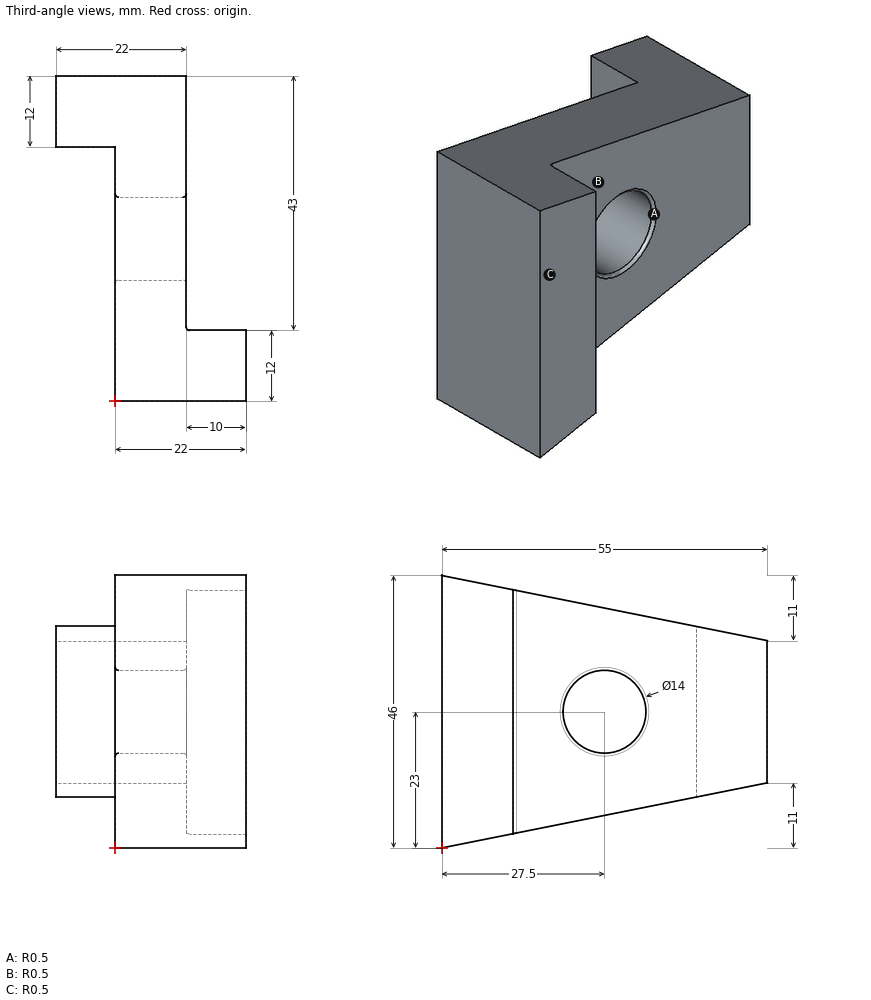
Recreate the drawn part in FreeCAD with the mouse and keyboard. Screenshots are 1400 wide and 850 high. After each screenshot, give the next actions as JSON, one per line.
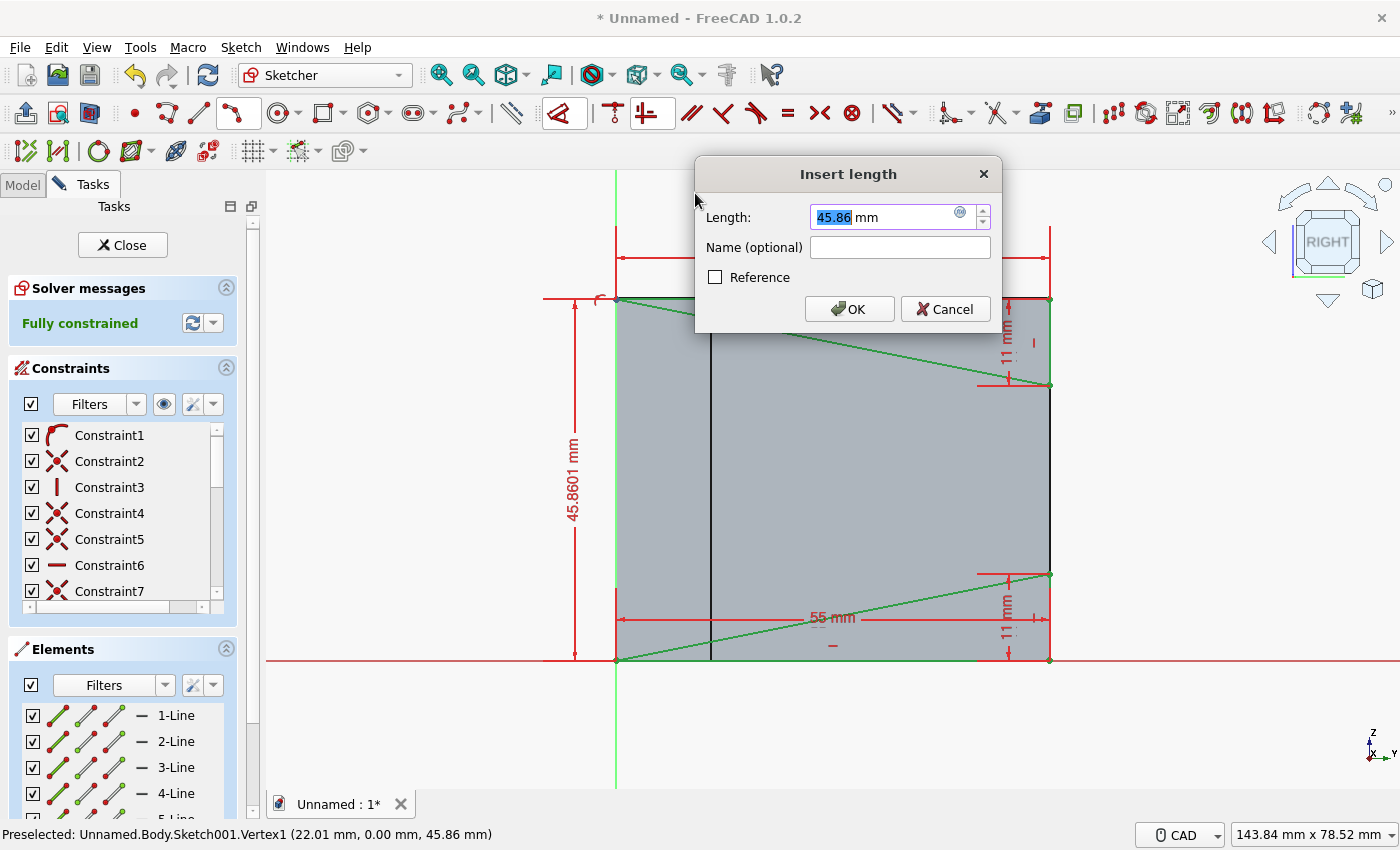
{"action": "type", "text": "46"}
{"action": "key", "text": "Return"}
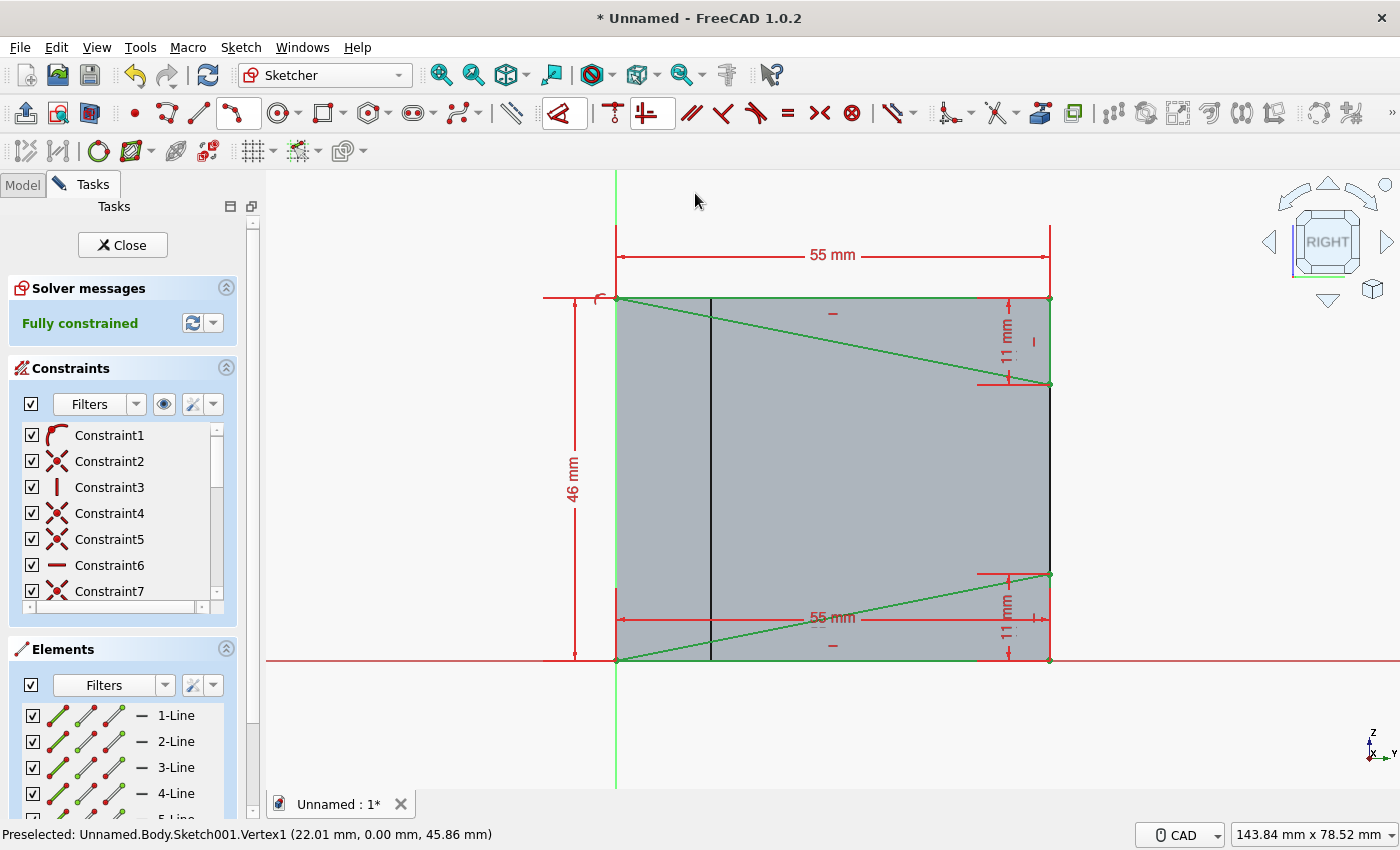
{"action": "left_click", "coordinate": [123, 245]}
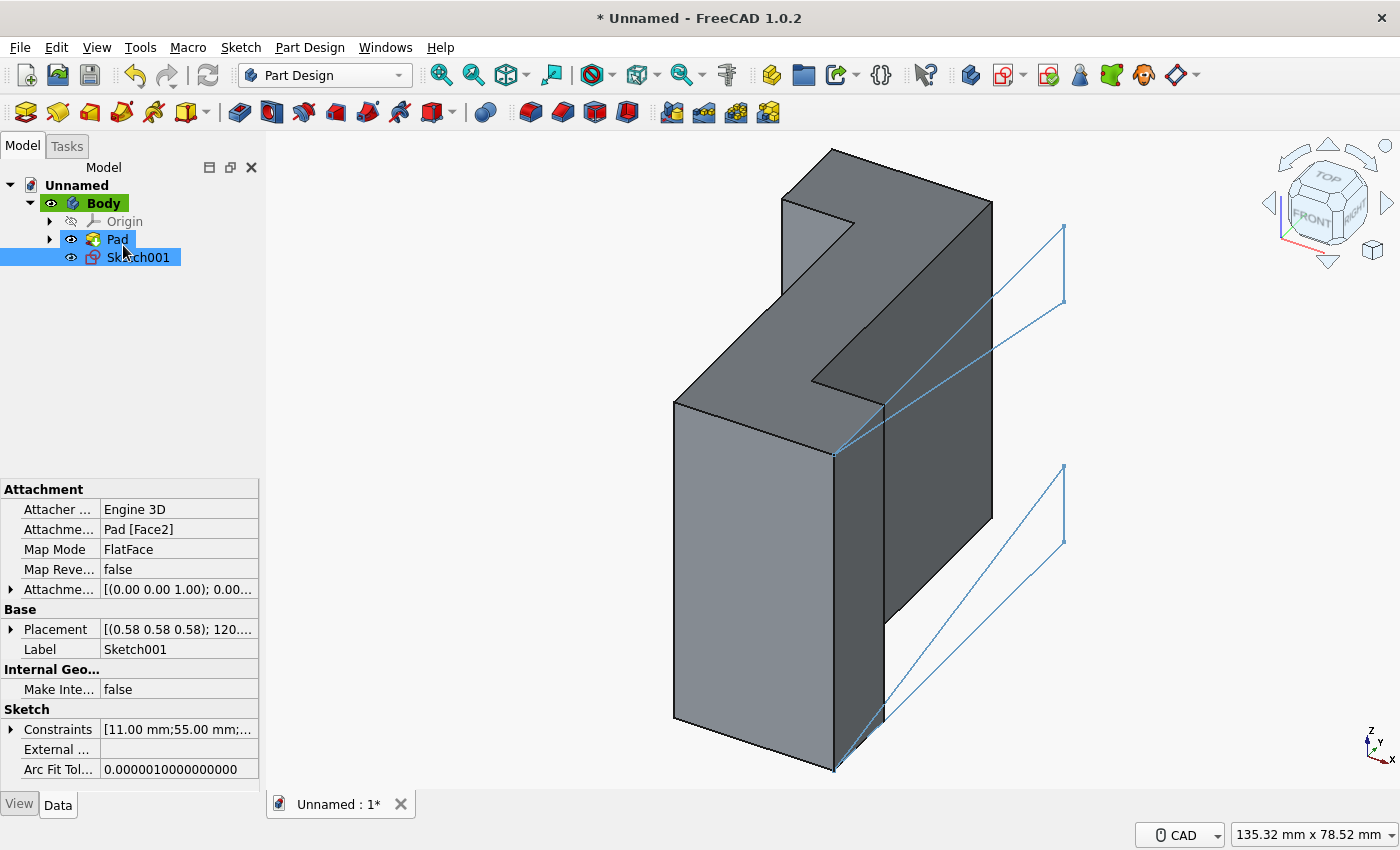
{"action": "left_click", "coordinate": [240, 112]}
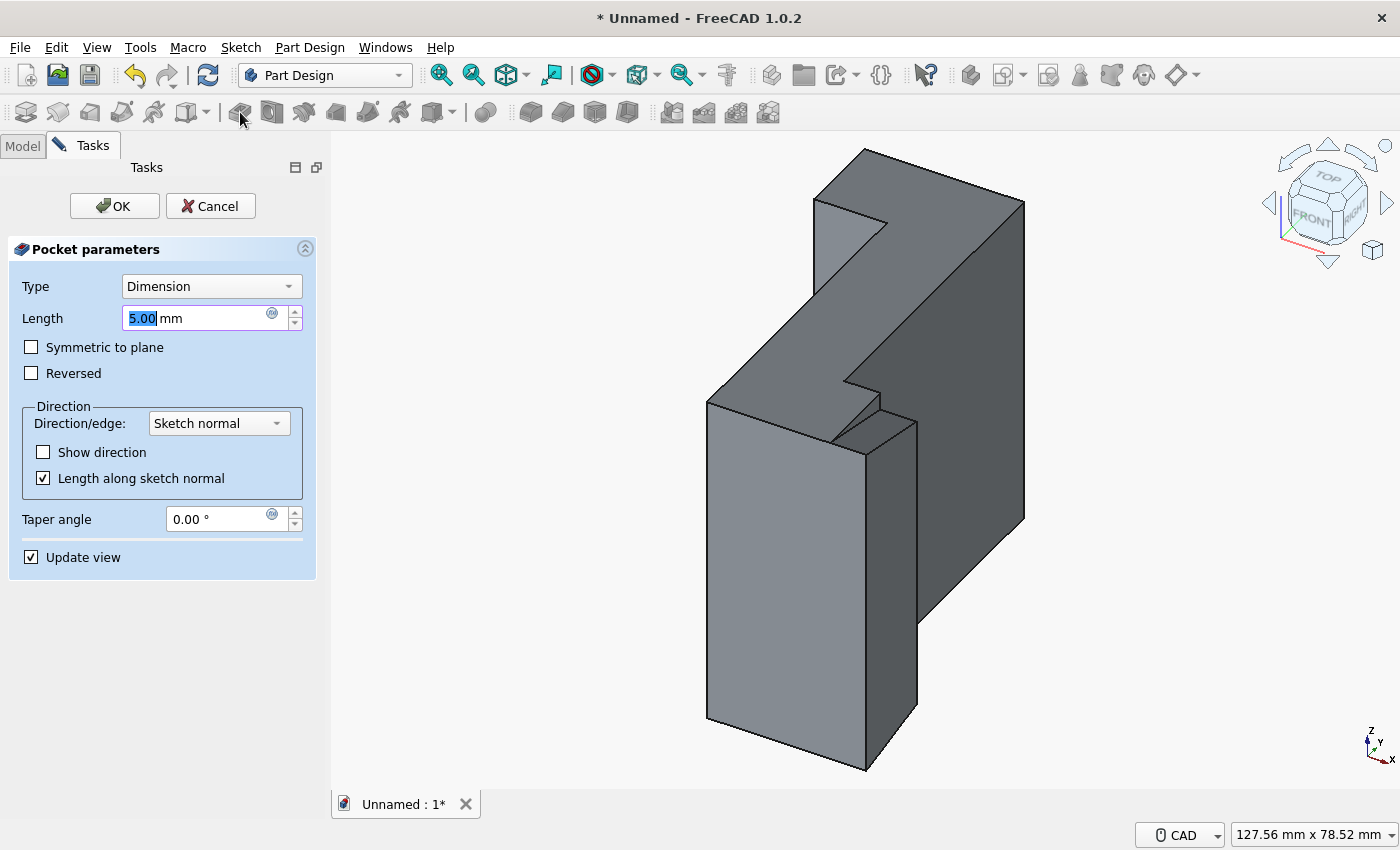
{"action": "type", "text": "46"}
{"action": "key", "text": "Tab"}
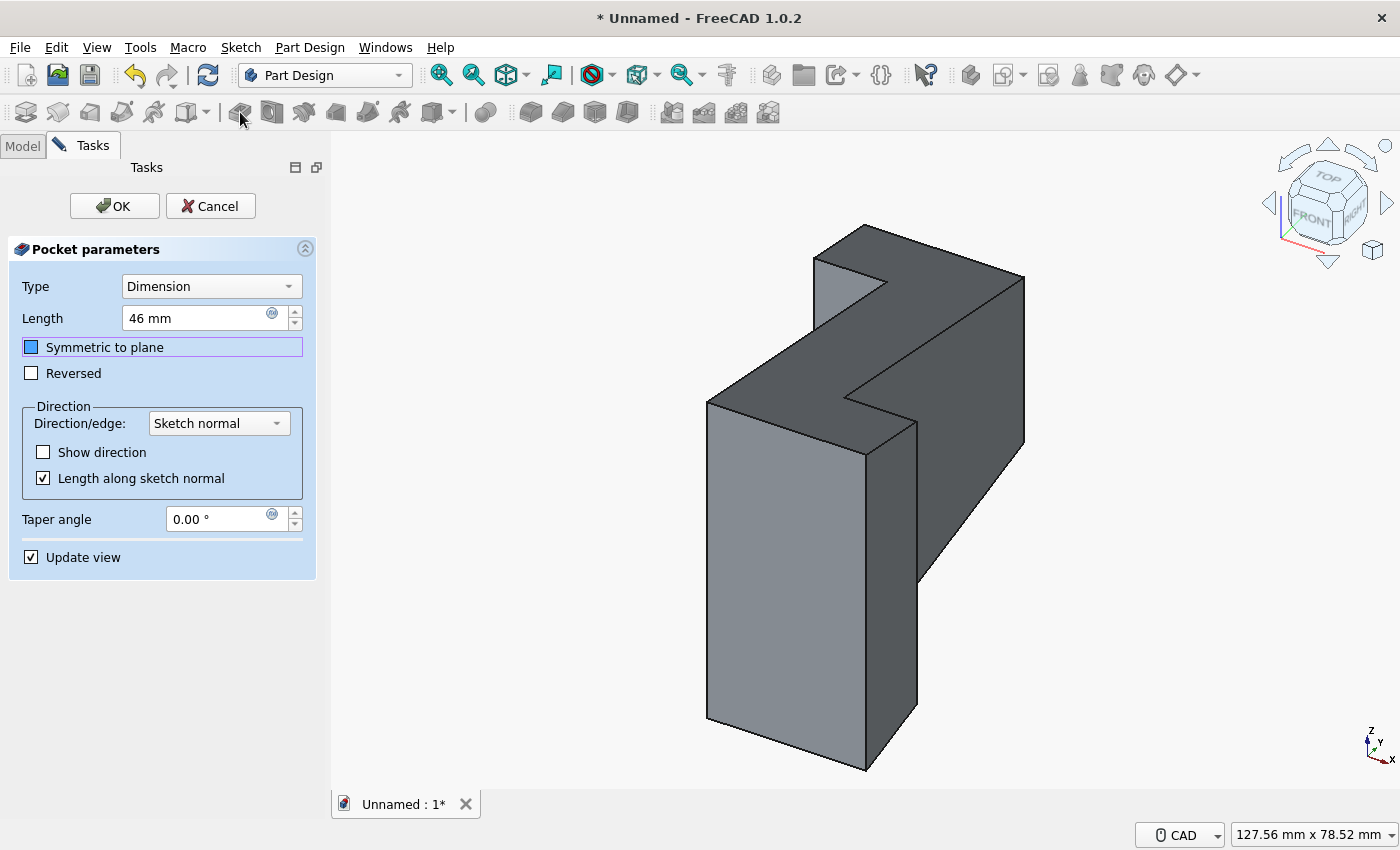
{"action": "left_click", "coordinate": [115, 206]}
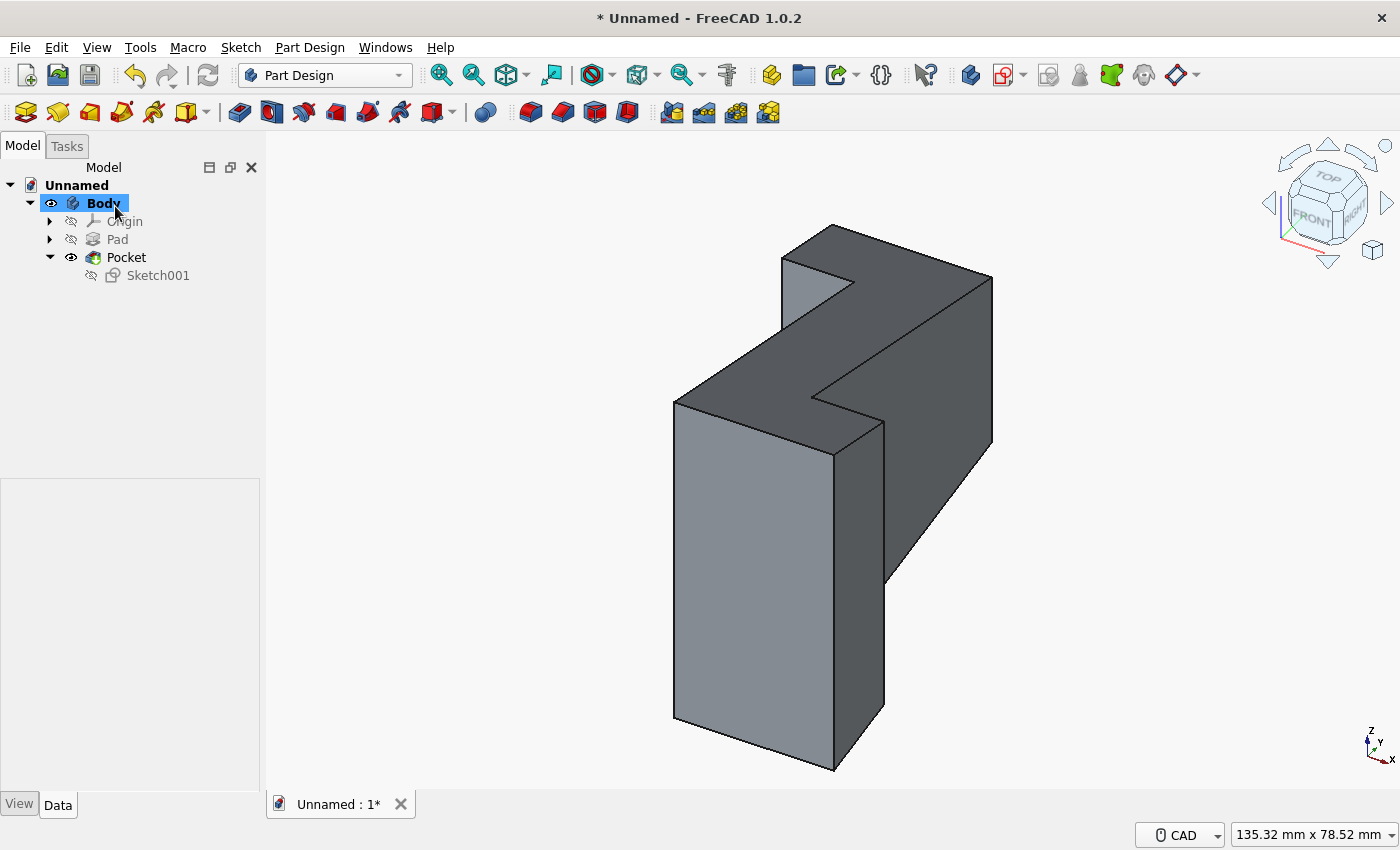
{"action": "key", "text": "6"}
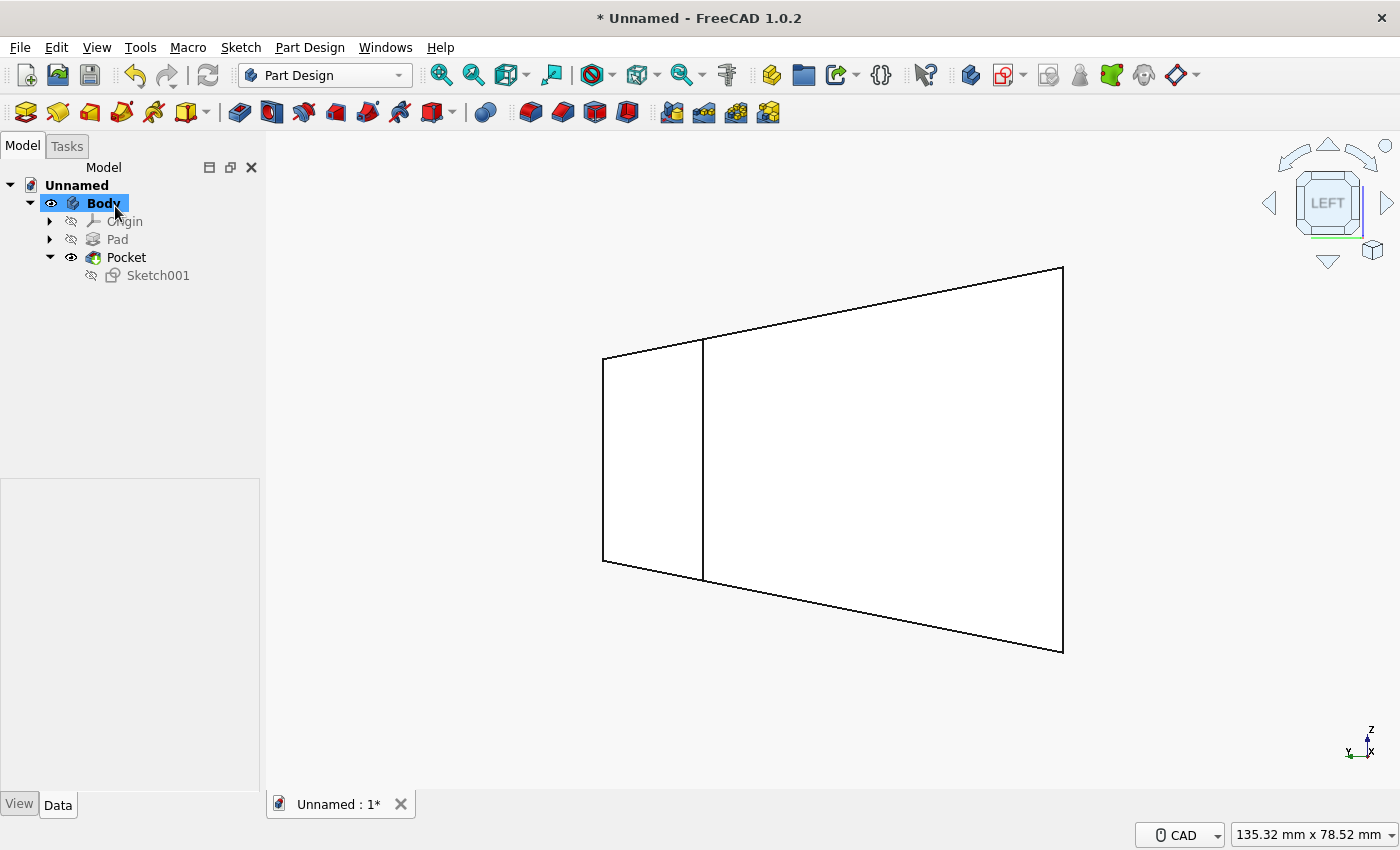
{"action": "left_click", "coordinate": [883, 459]}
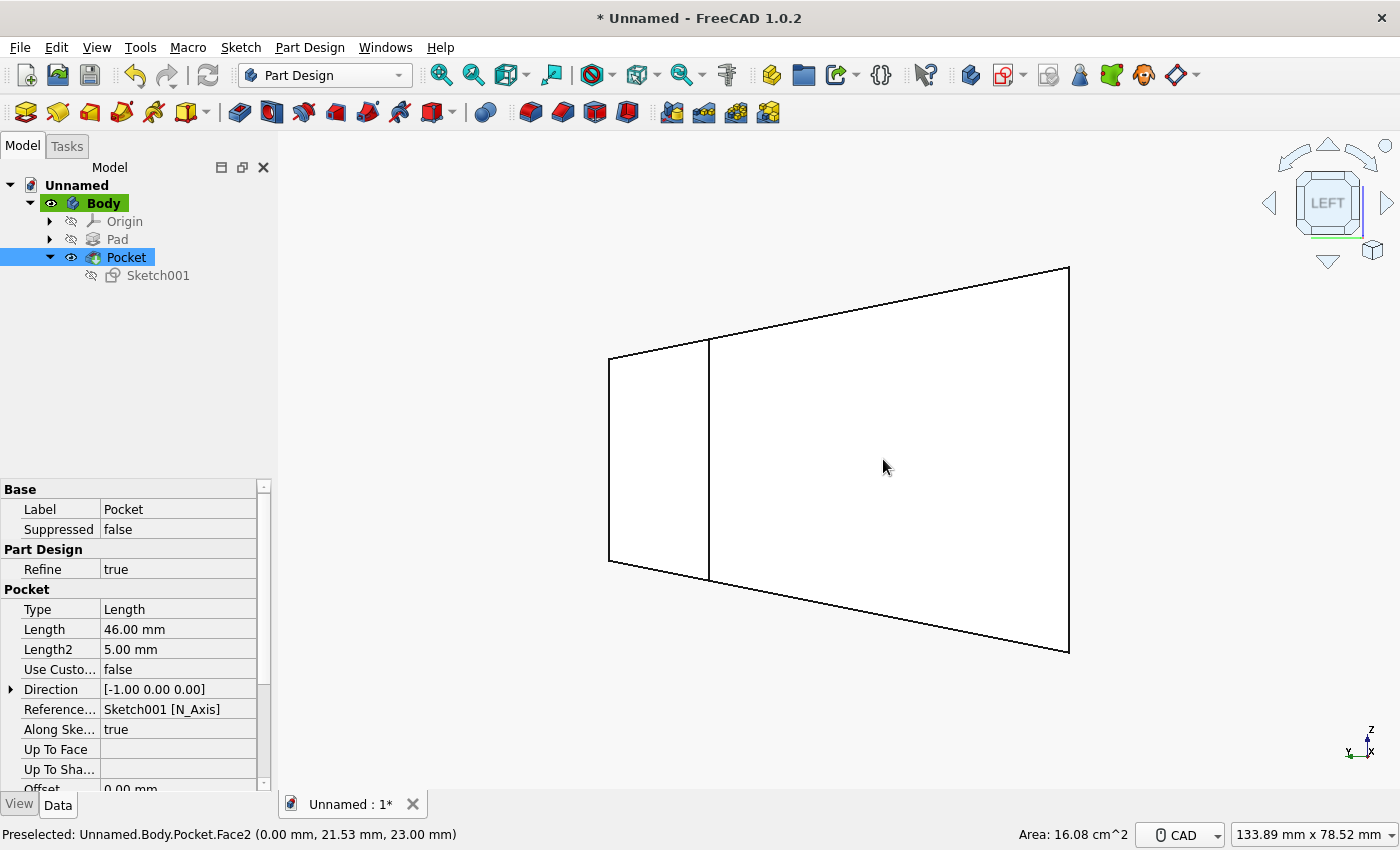
{"action": "left_click", "coordinate": [1004, 76]}